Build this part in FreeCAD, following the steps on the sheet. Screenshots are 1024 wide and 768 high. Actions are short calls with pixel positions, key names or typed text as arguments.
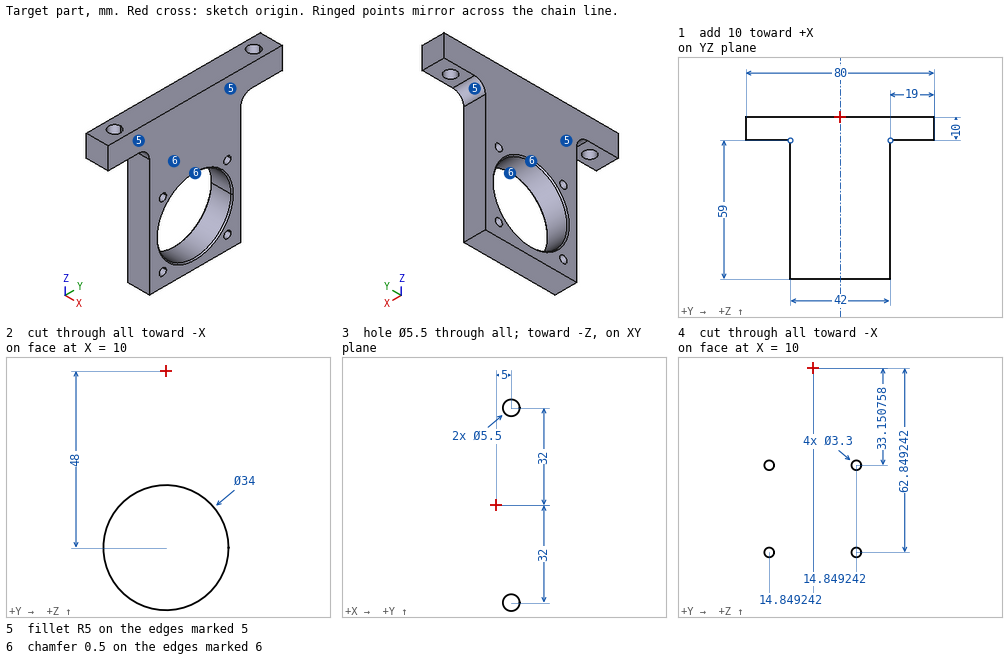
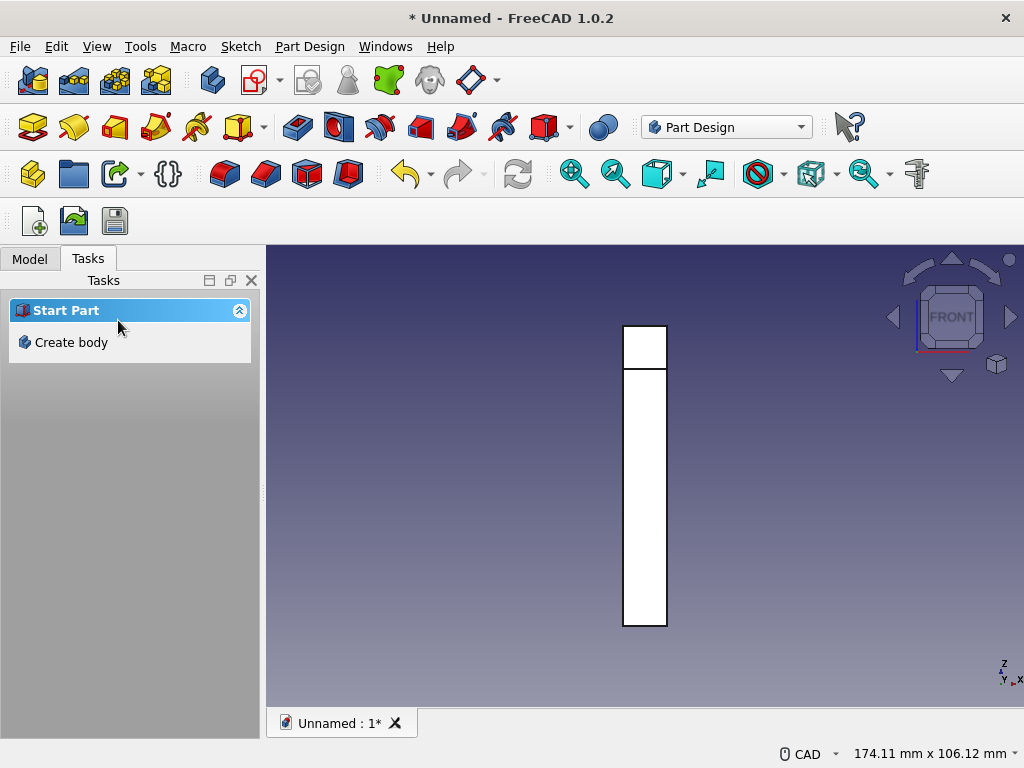
key(3)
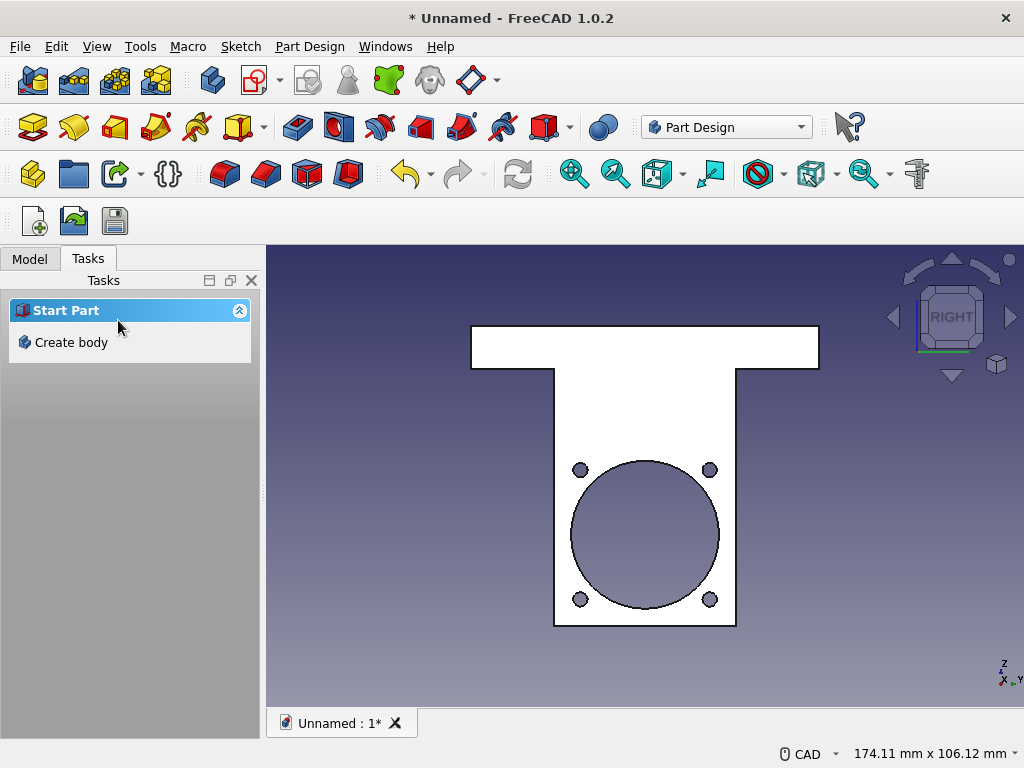
key(5)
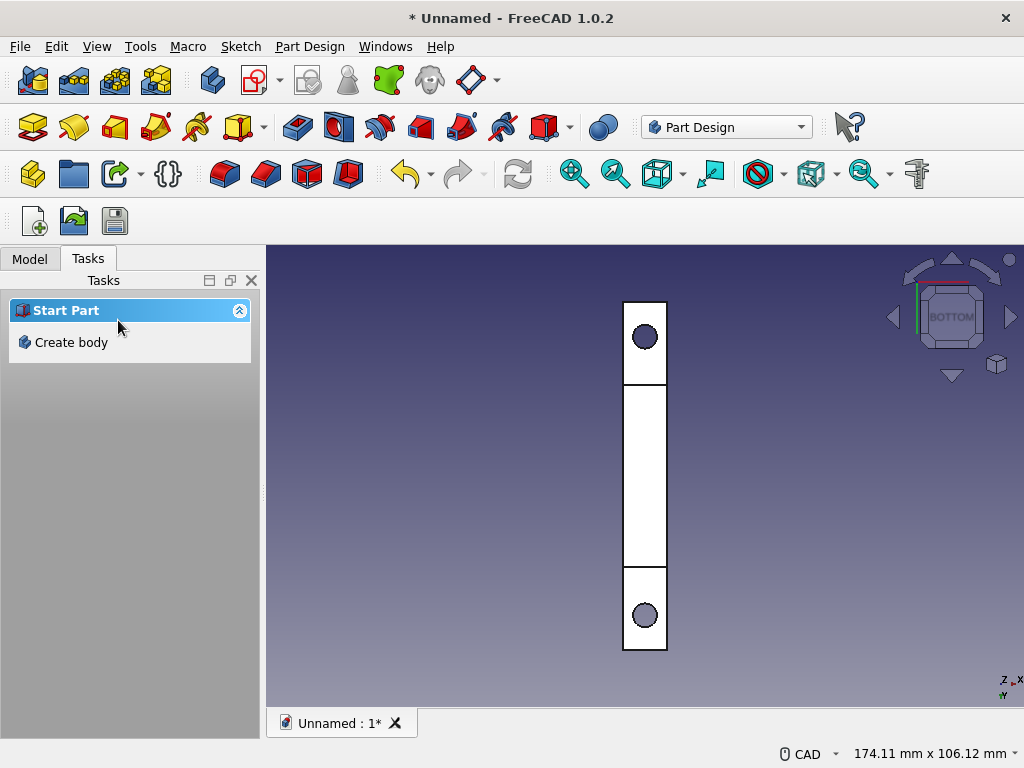
key(4)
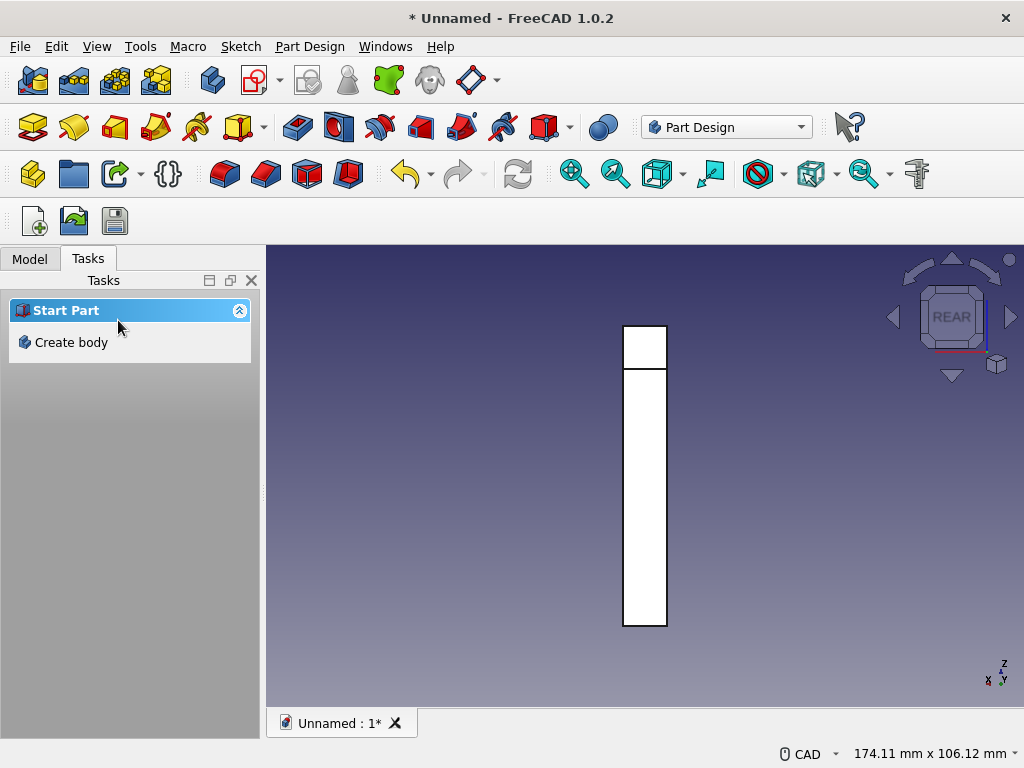
key(6)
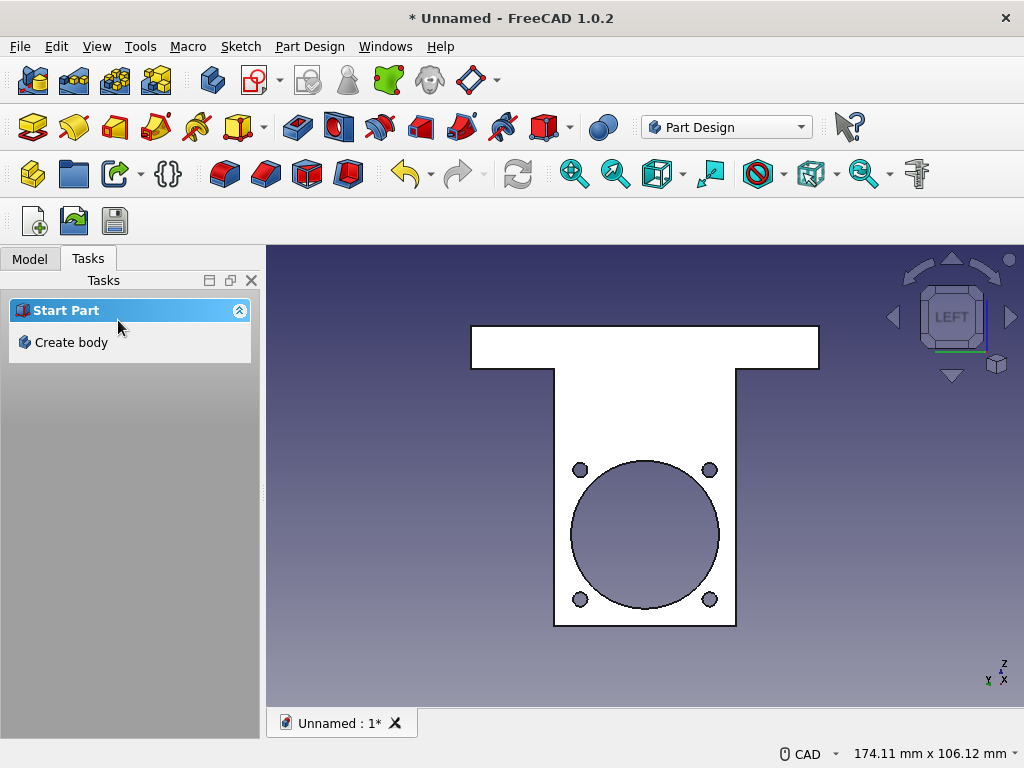
key(v)
key(3)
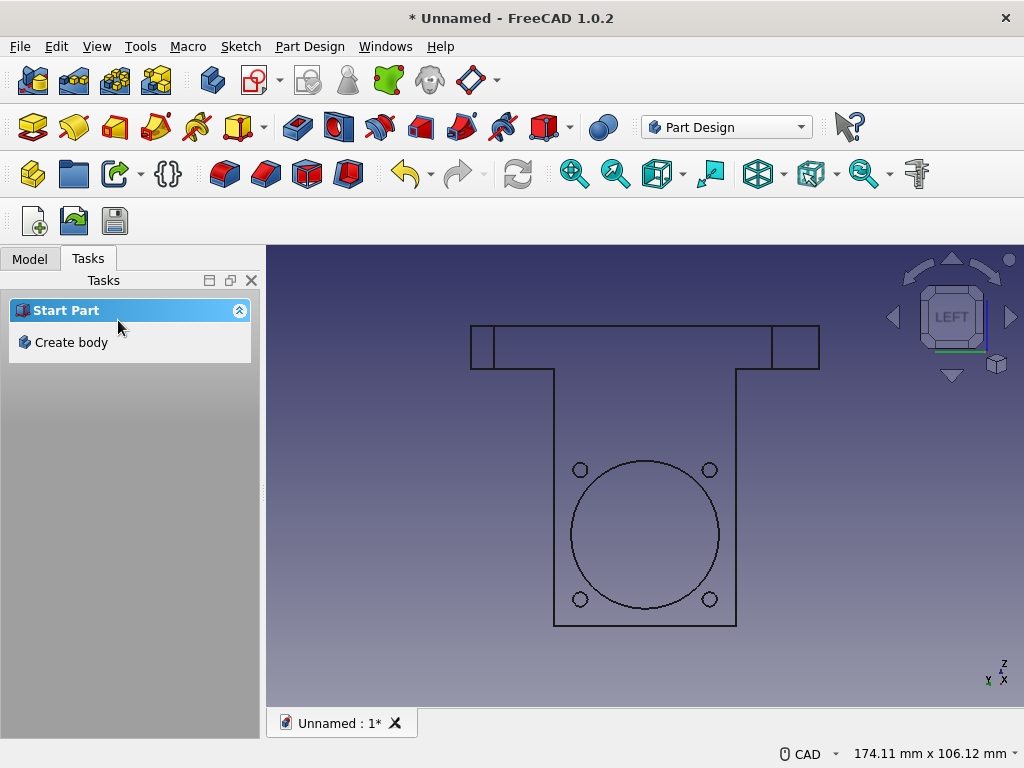
key(0)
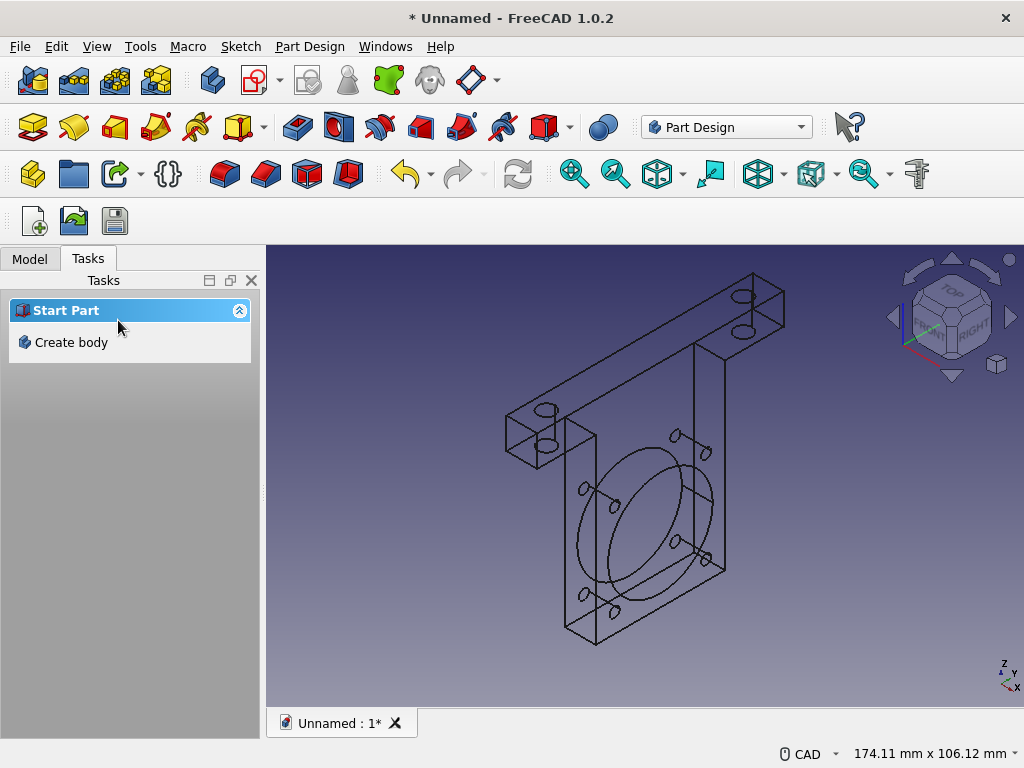
click(710, 351)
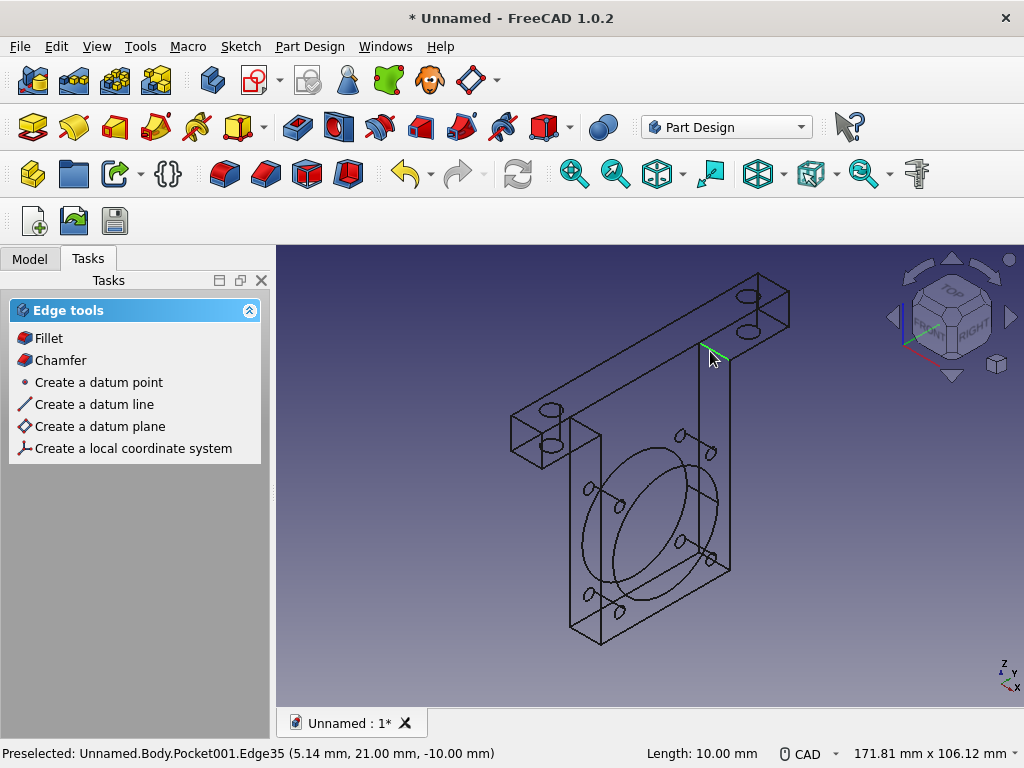
click(585, 425, ctrl)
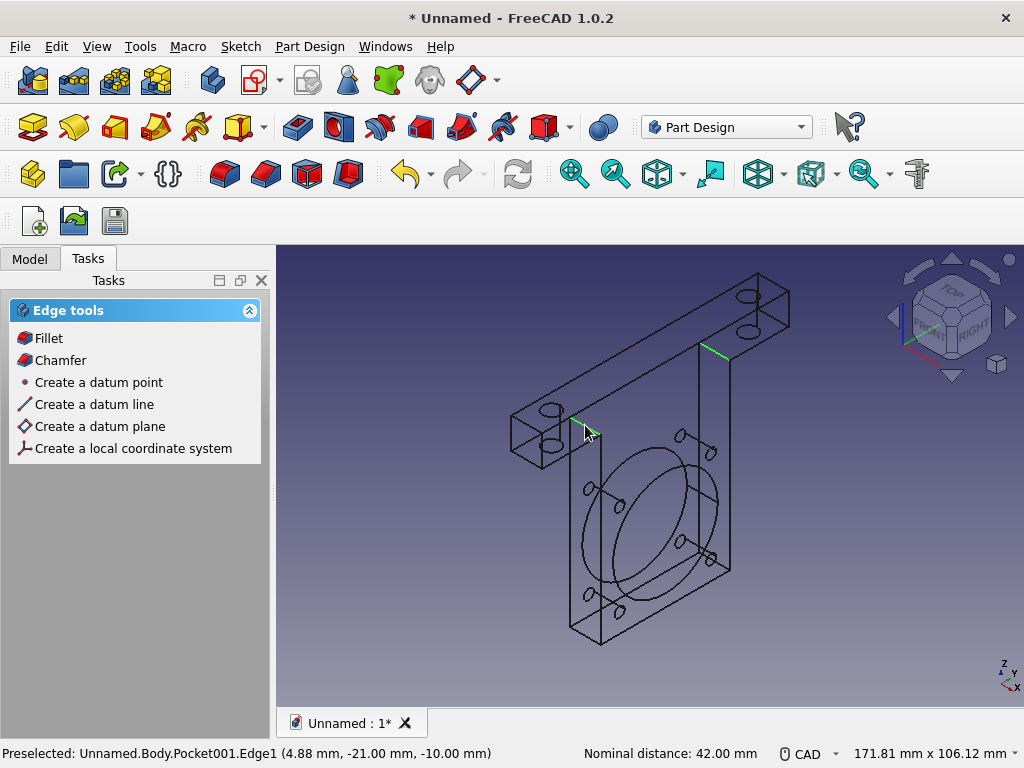
key(v)
key(1)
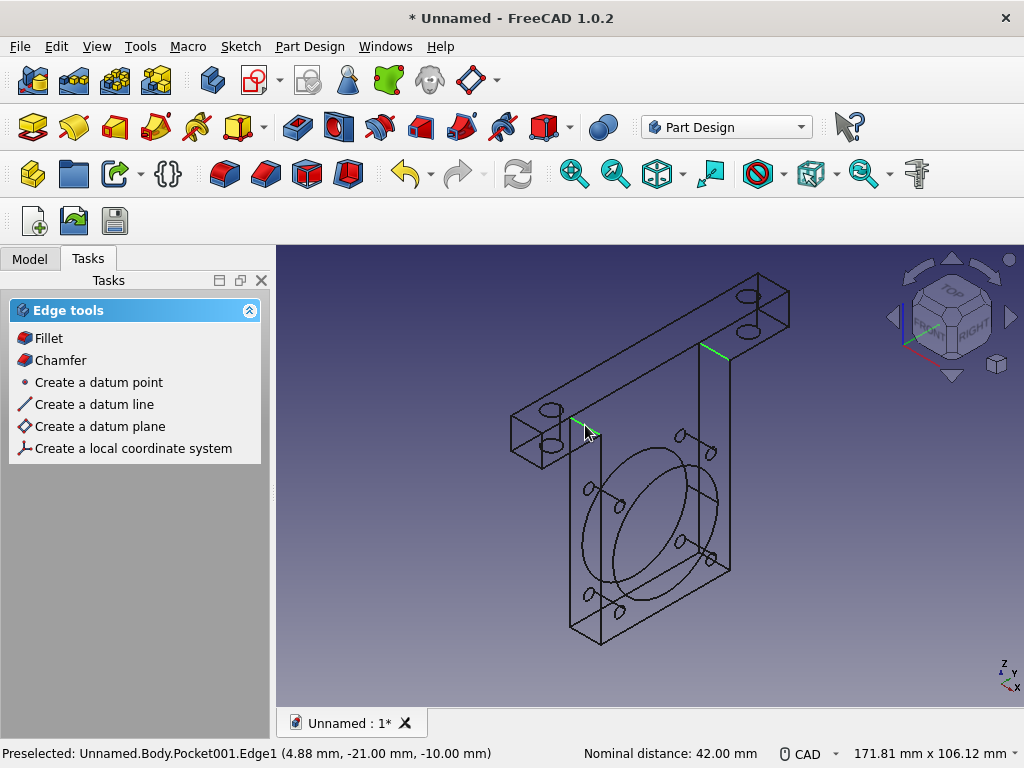
click(225, 174)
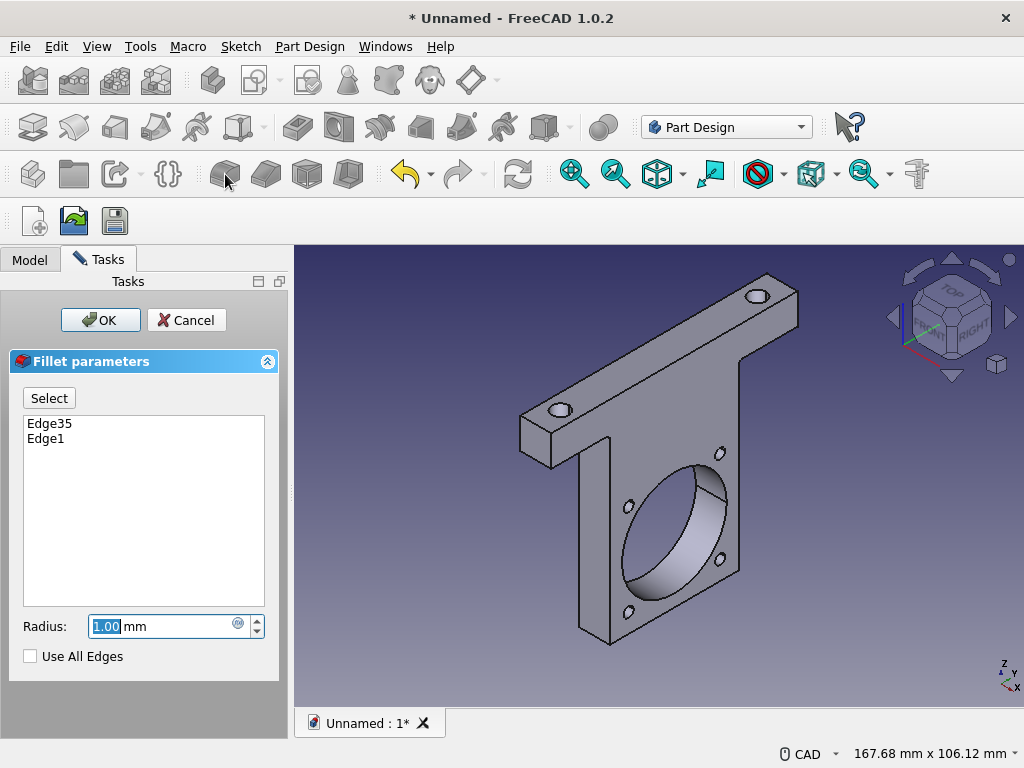
text(5)
key(Tab)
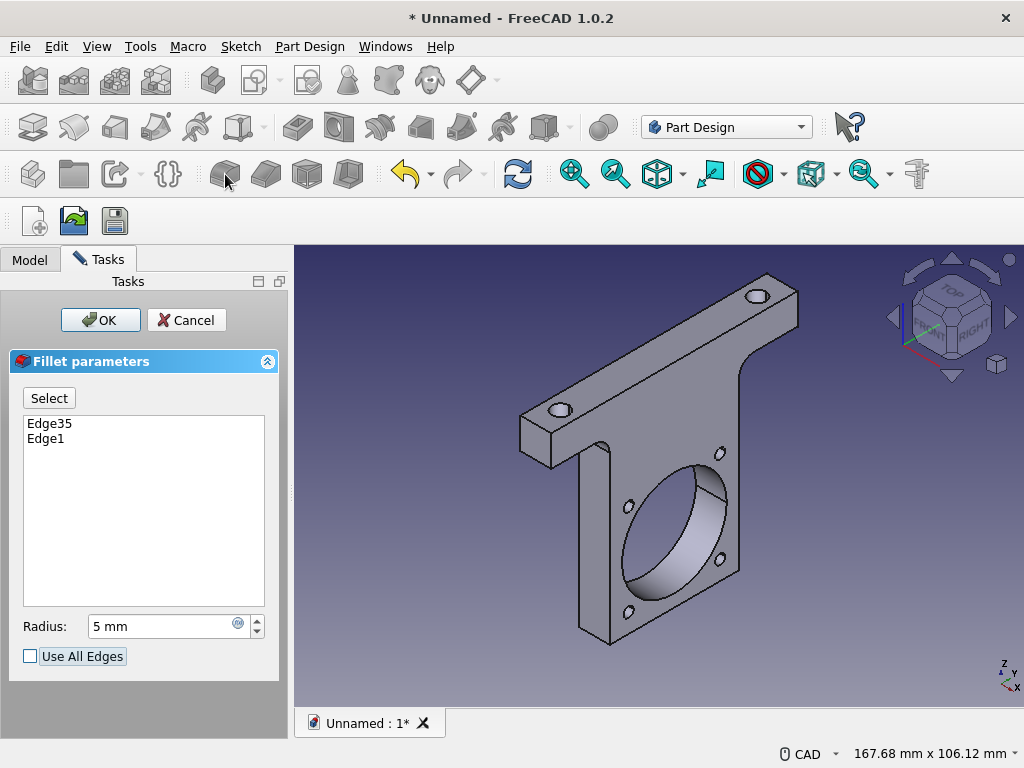
click(101, 320)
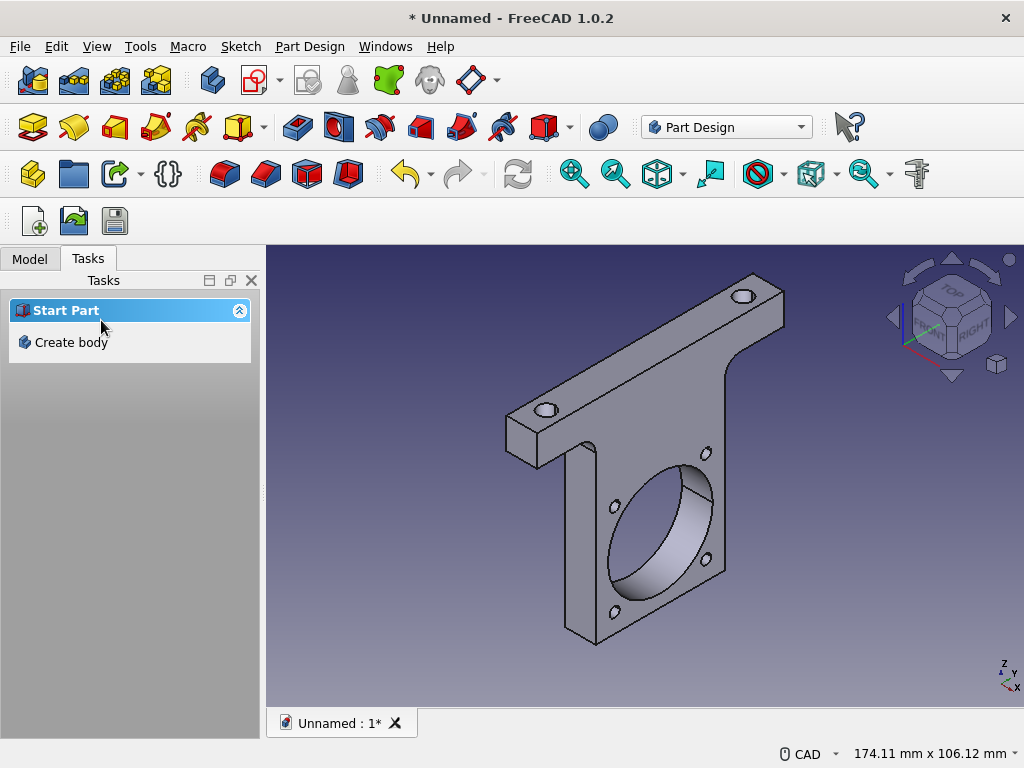
click(644, 599)